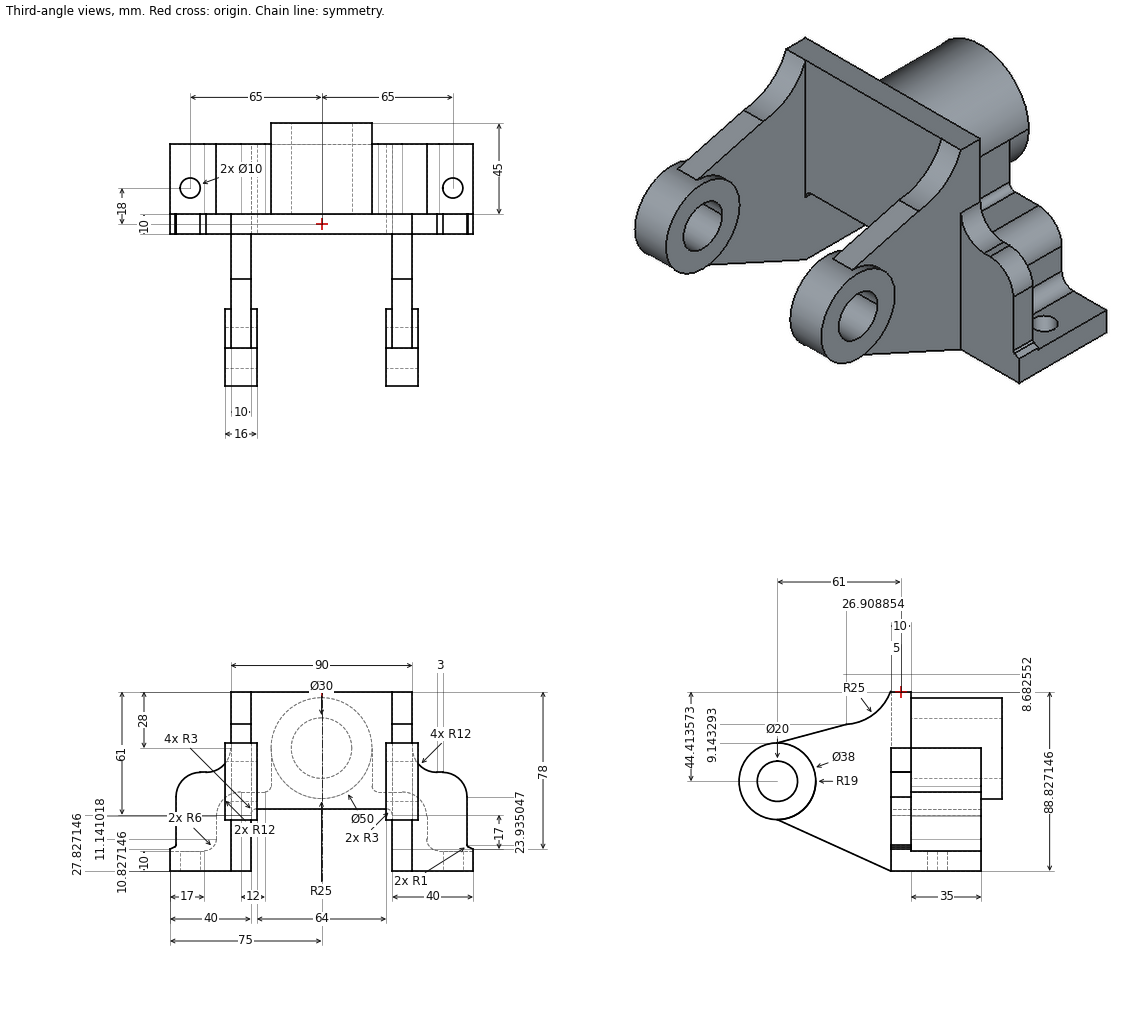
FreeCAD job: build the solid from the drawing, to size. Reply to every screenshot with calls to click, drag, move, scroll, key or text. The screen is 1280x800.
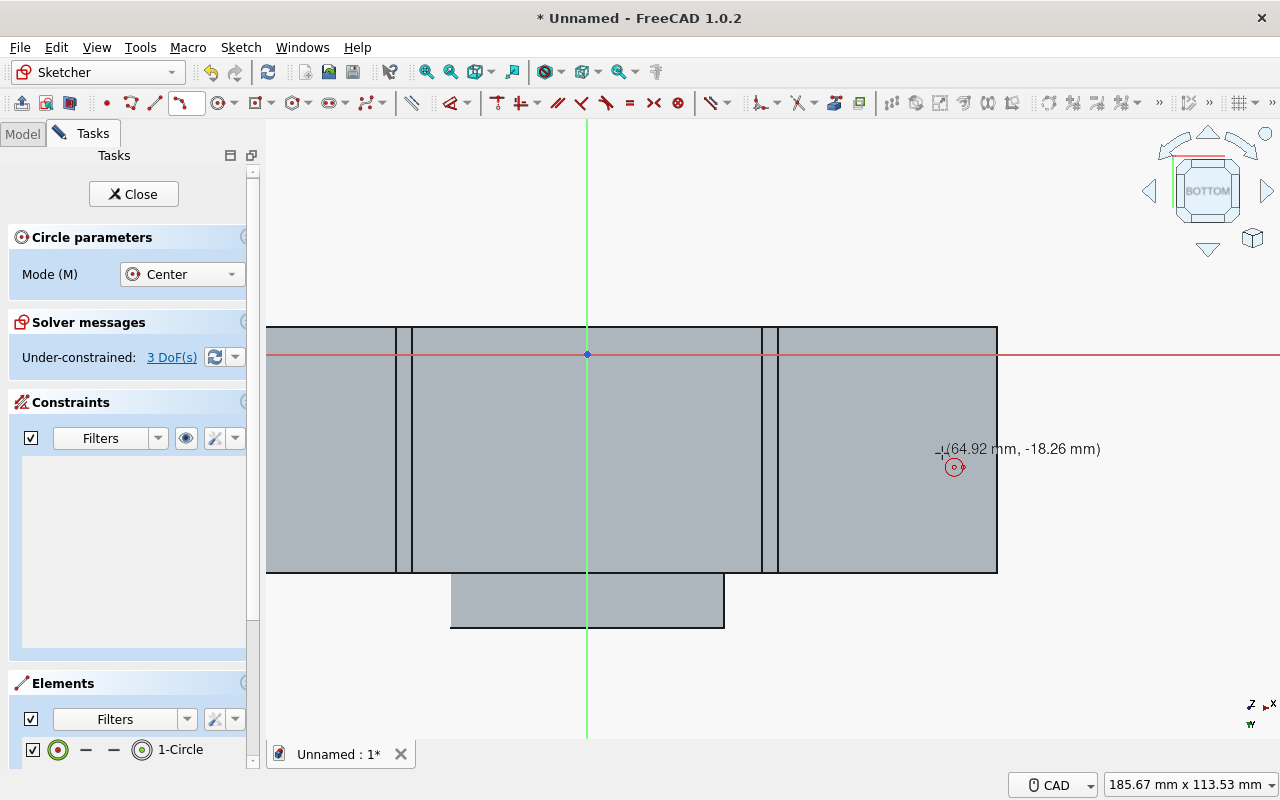
click(942, 453)
click(961, 434)
key(Escape)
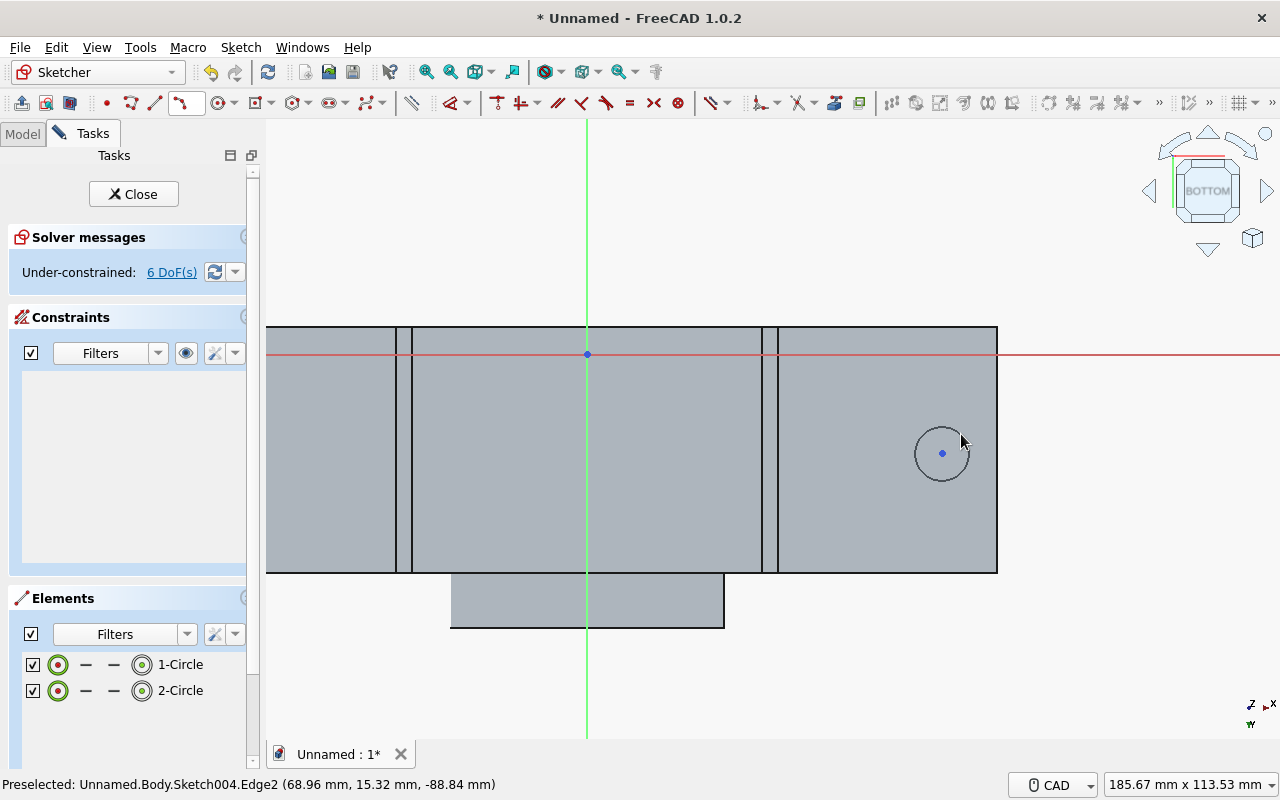
scroll(1115, 482, down, 1)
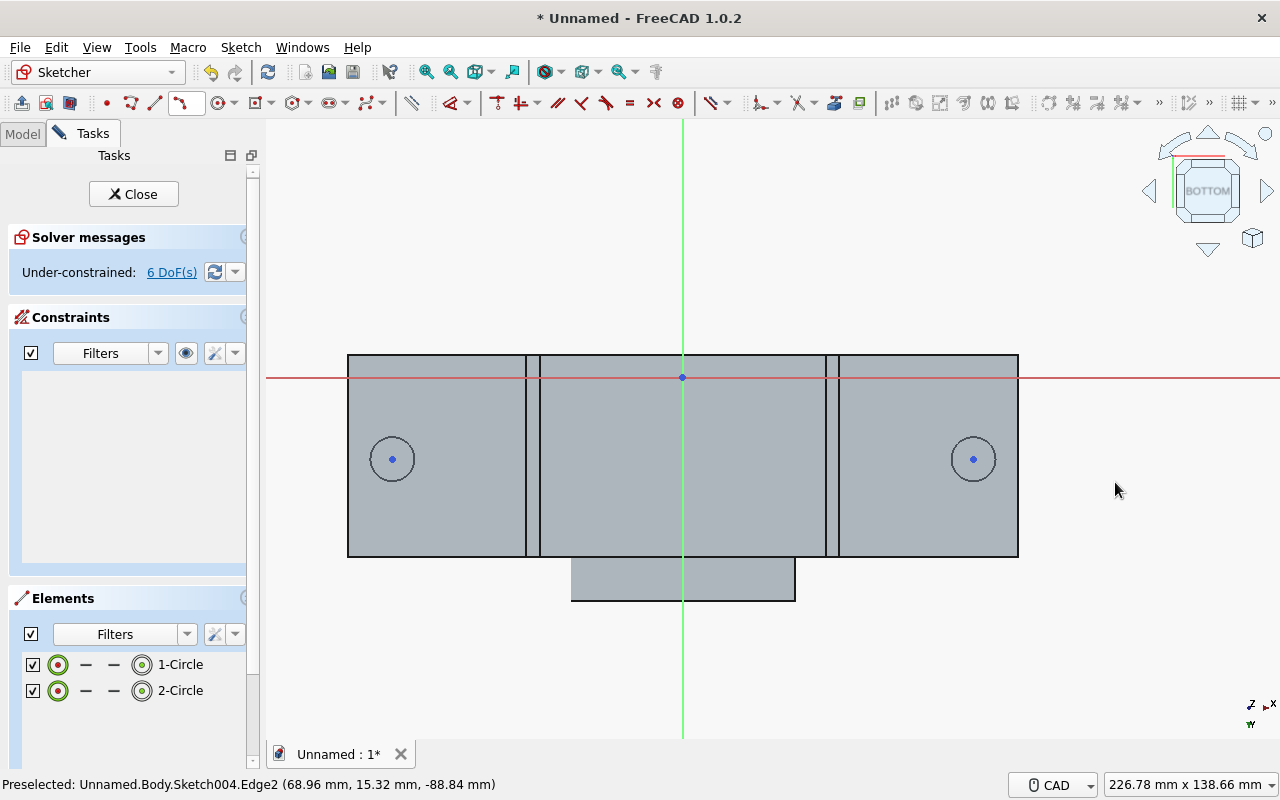
click(408, 444)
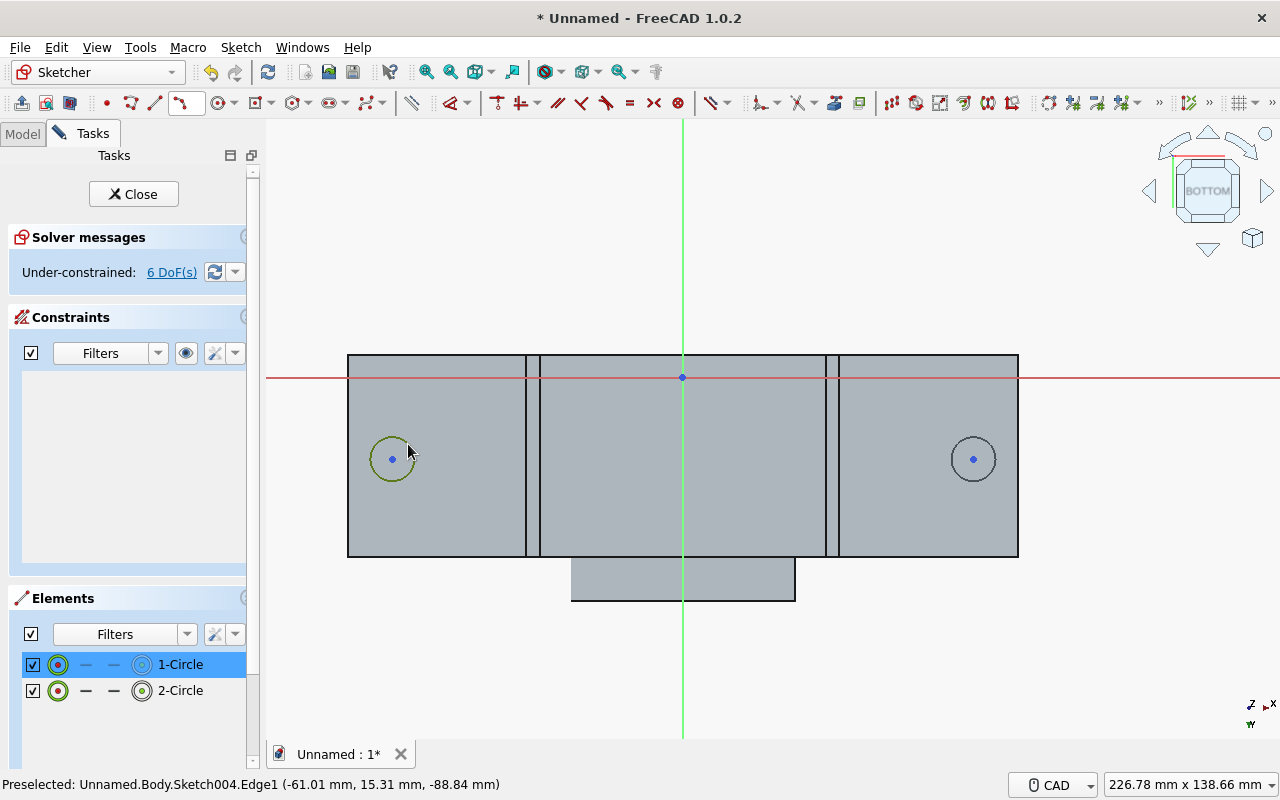
click(989, 444)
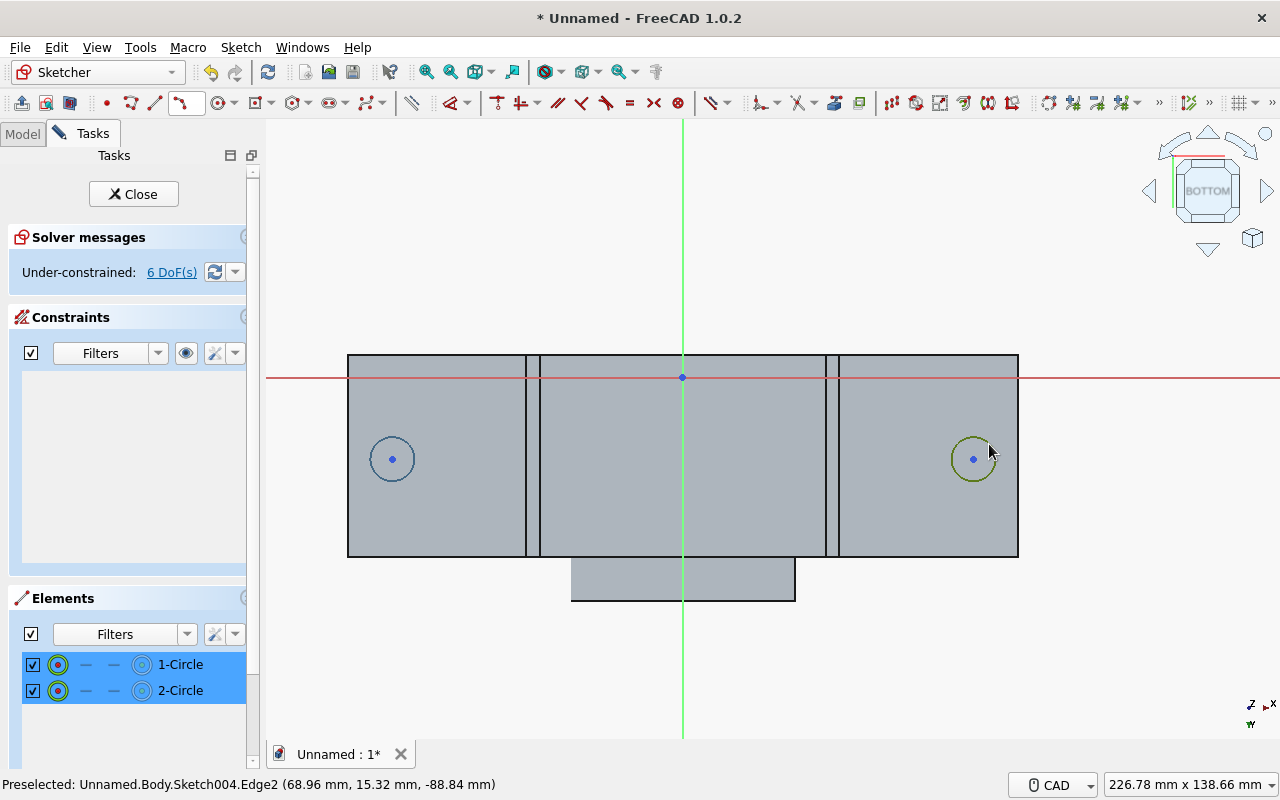
key(e)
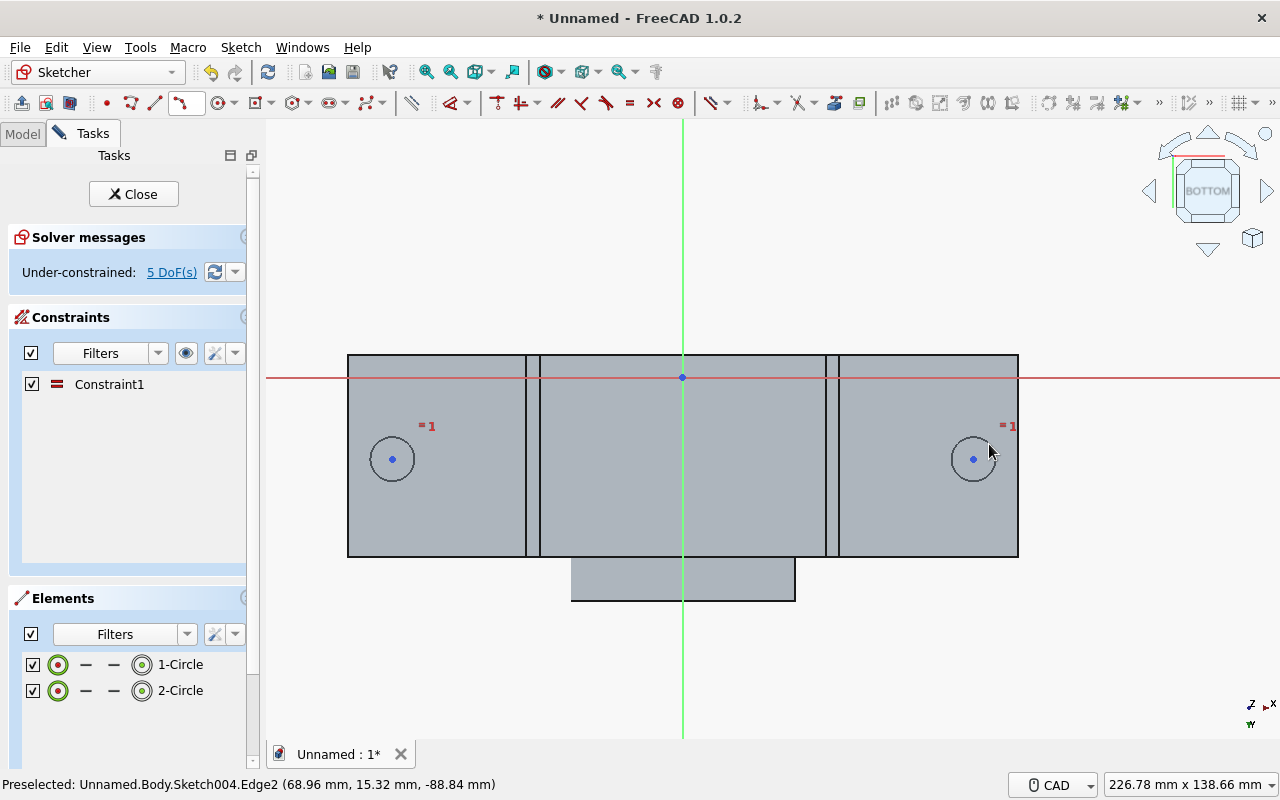
click(392, 459)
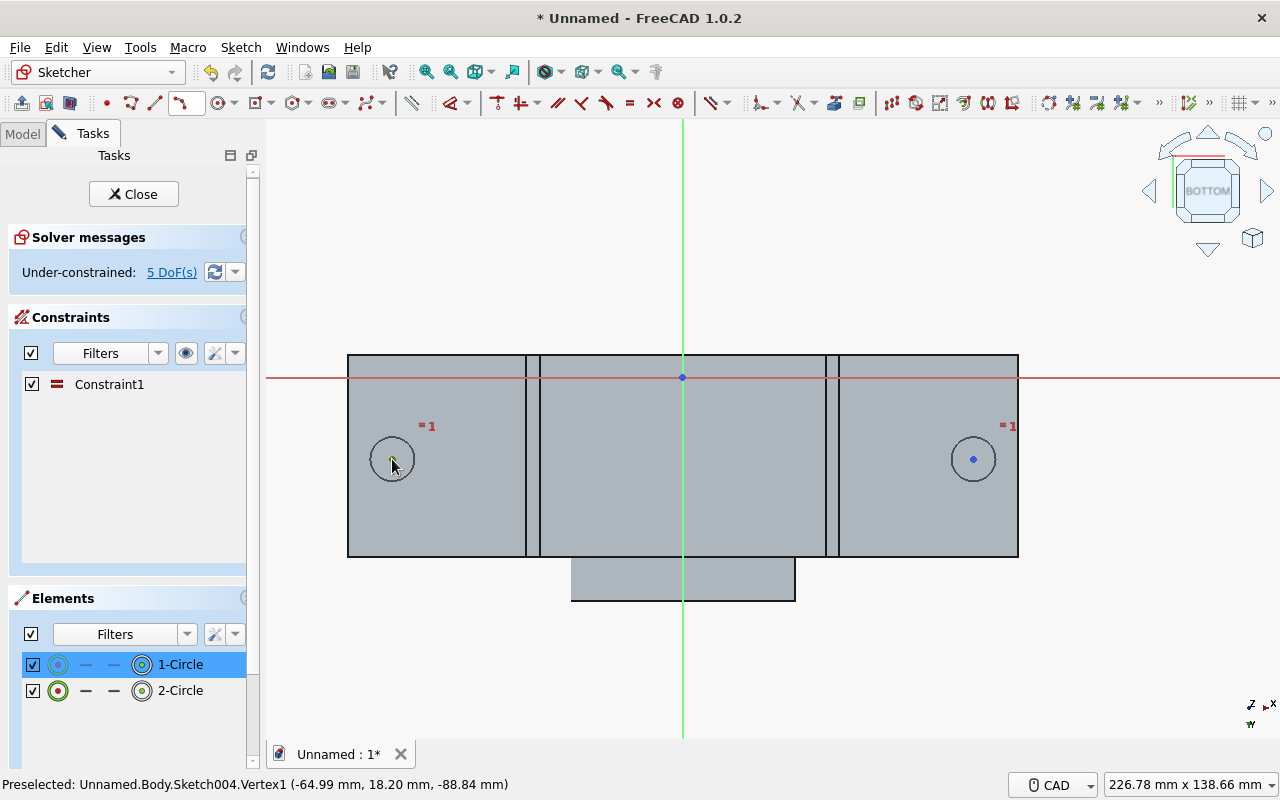
click(974, 459)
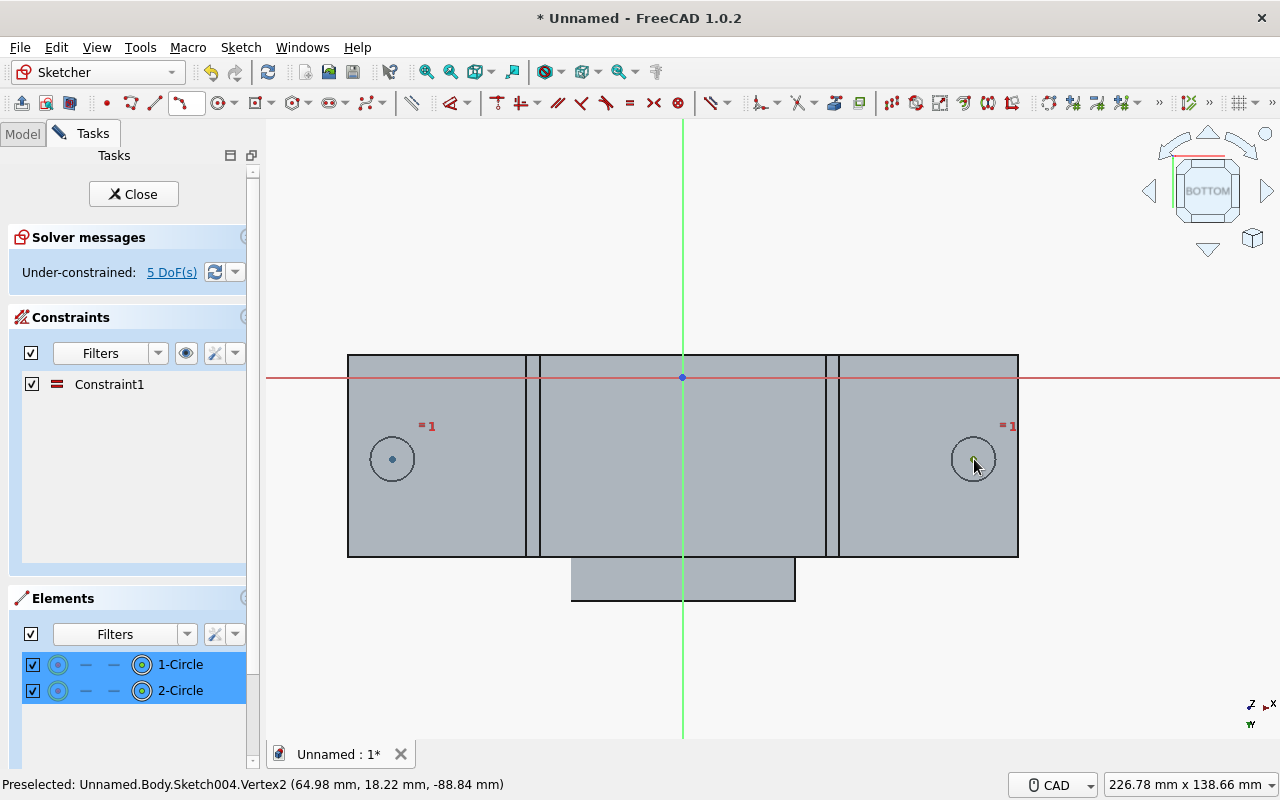
key(h)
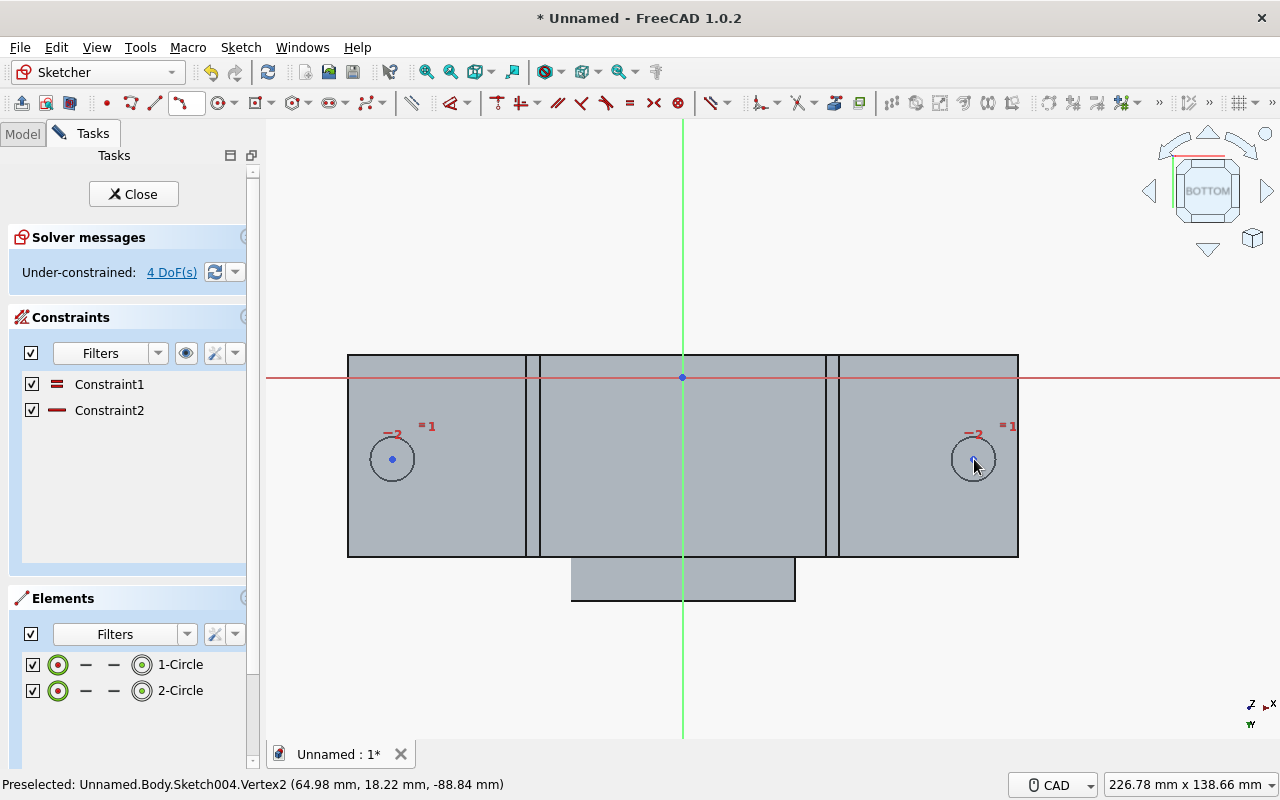
key(d)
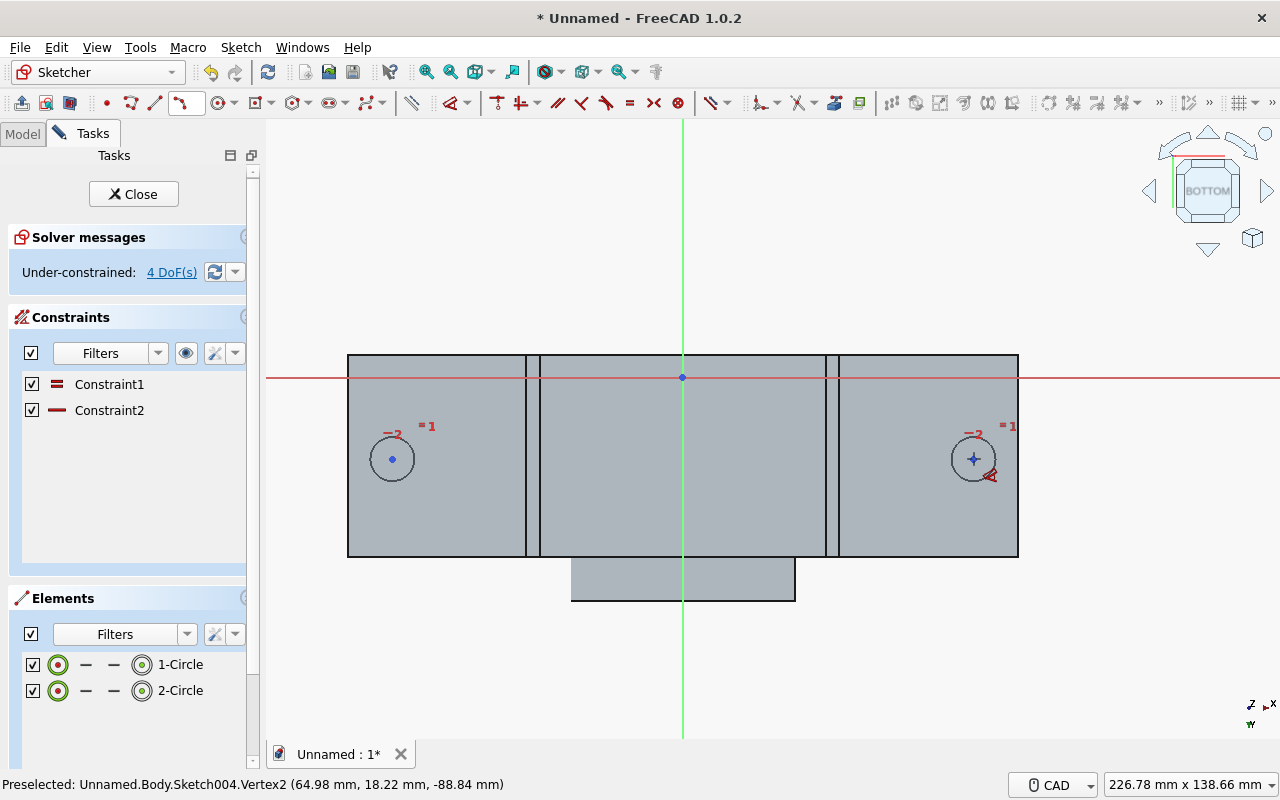
click(408, 444)
click(431, 422)